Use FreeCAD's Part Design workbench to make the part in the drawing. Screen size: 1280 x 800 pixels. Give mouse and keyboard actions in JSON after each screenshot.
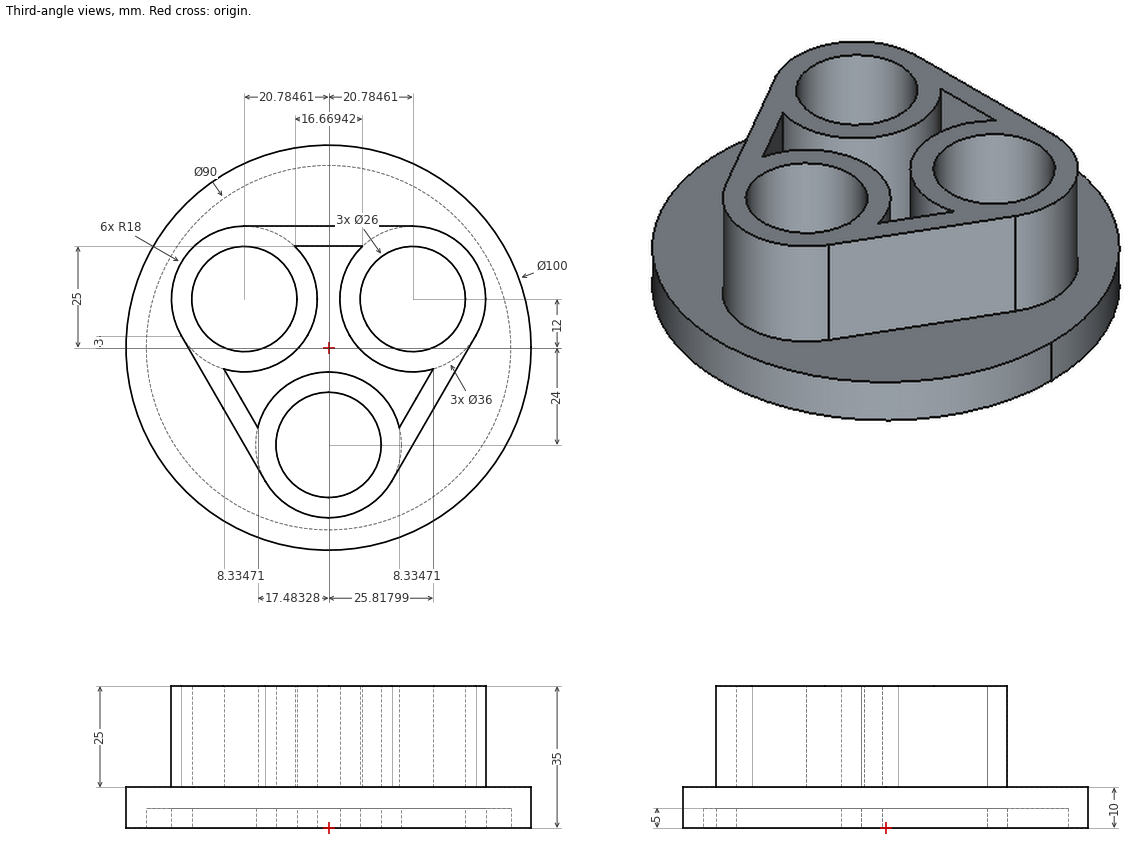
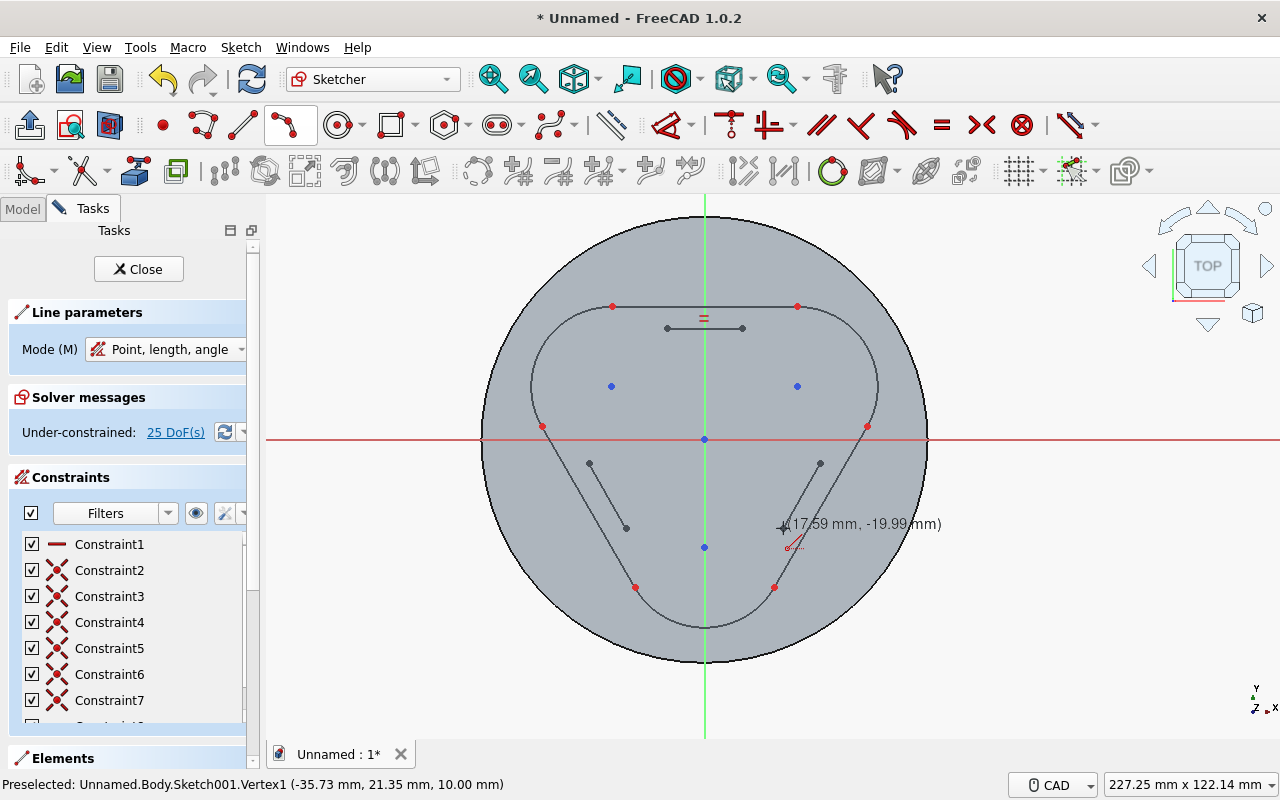
{"action": "left_click", "coordinate": [284, 126]}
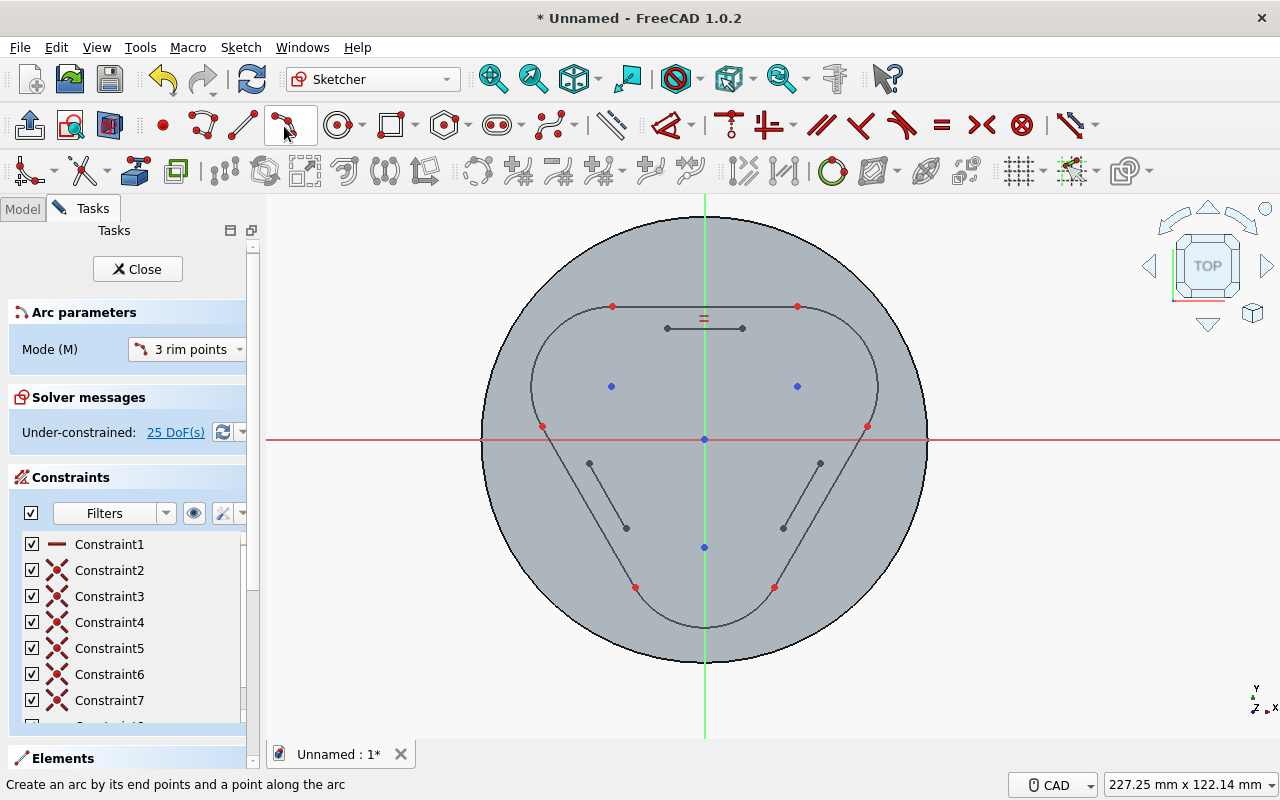
{"action": "left_click", "coordinate": [589, 464]}
{"action": "left_click", "coordinate": [667, 329]}
{"action": "left_click", "coordinate": [689, 407]}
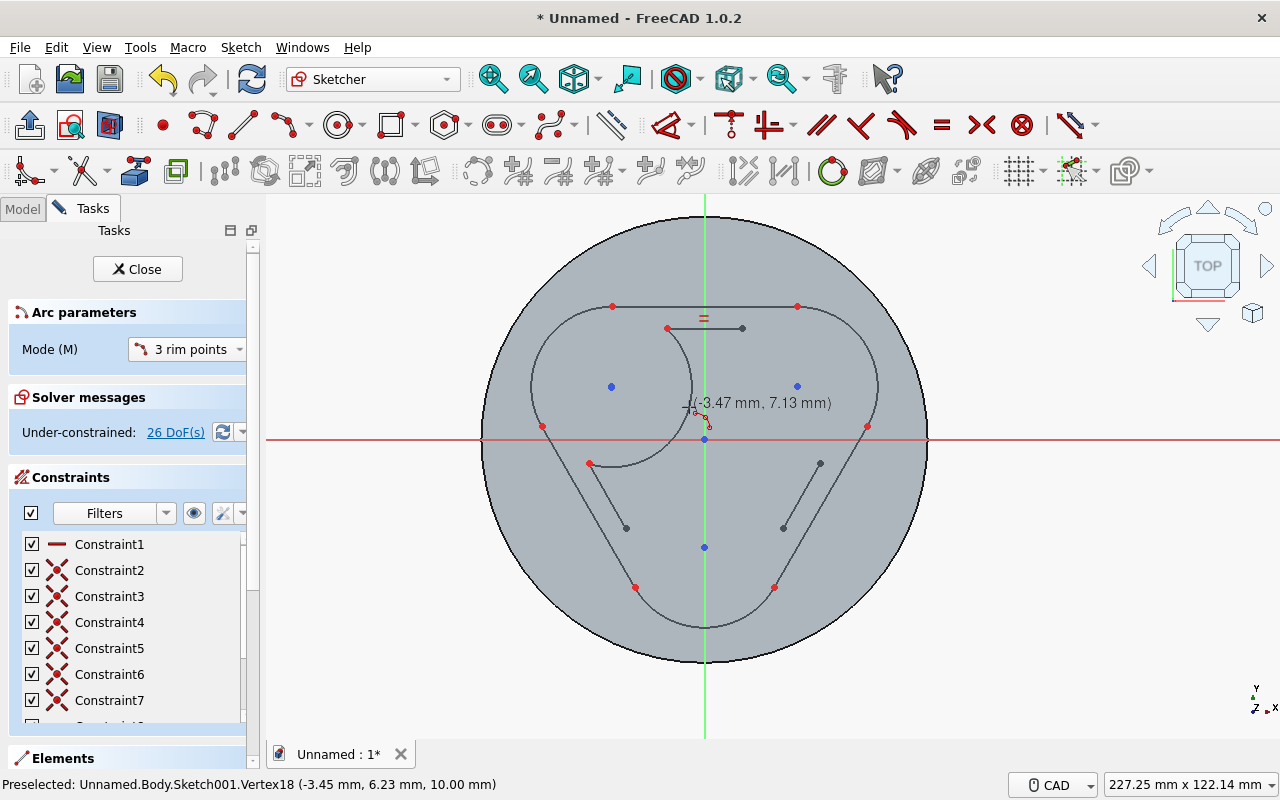
{"action": "left_click", "coordinate": [742, 329]}
{"action": "left_click", "coordinate": [820, 464]}
{"action": "left_click", "coordinate": [720, 407]}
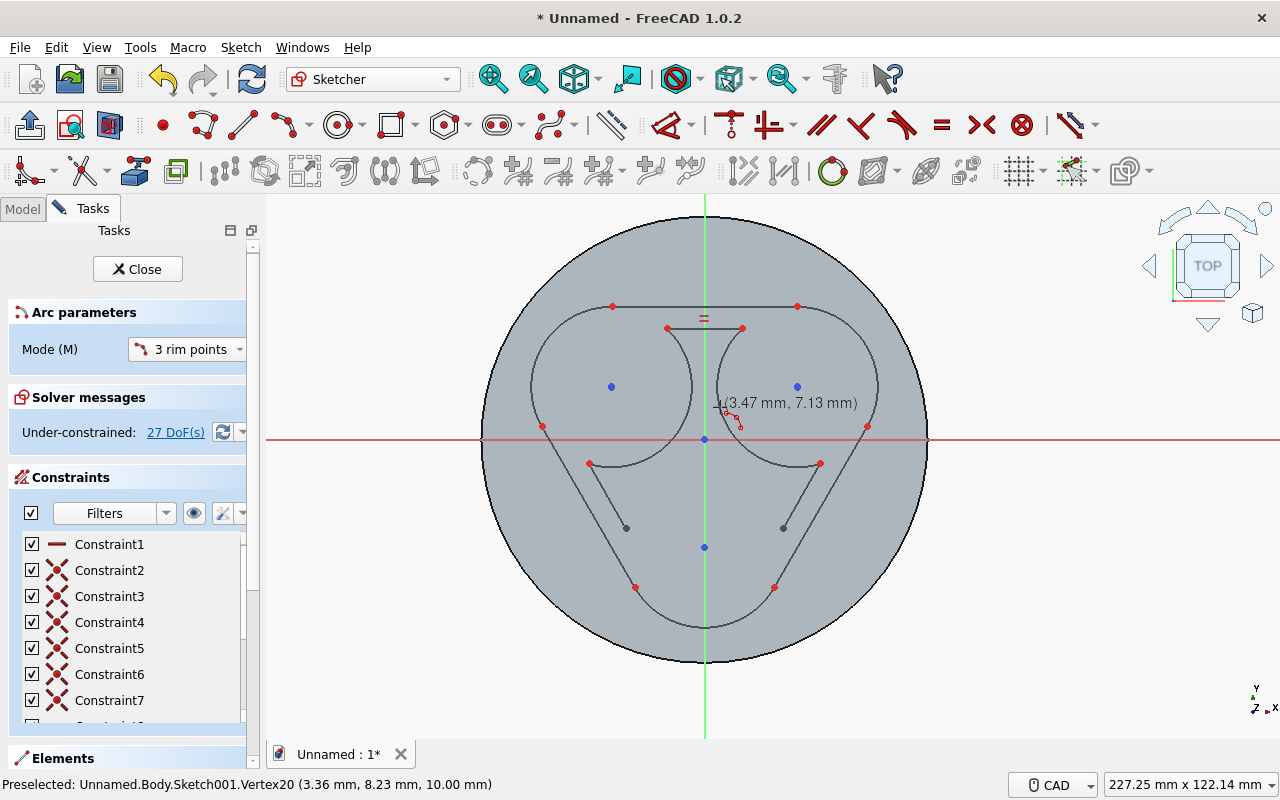
{"action": "left_click", "coordinate": [783, 529]}
{"action": "left_click", "coordinate": [626, 529]}
{"action": "left_click", "coordinate": [726, 469]}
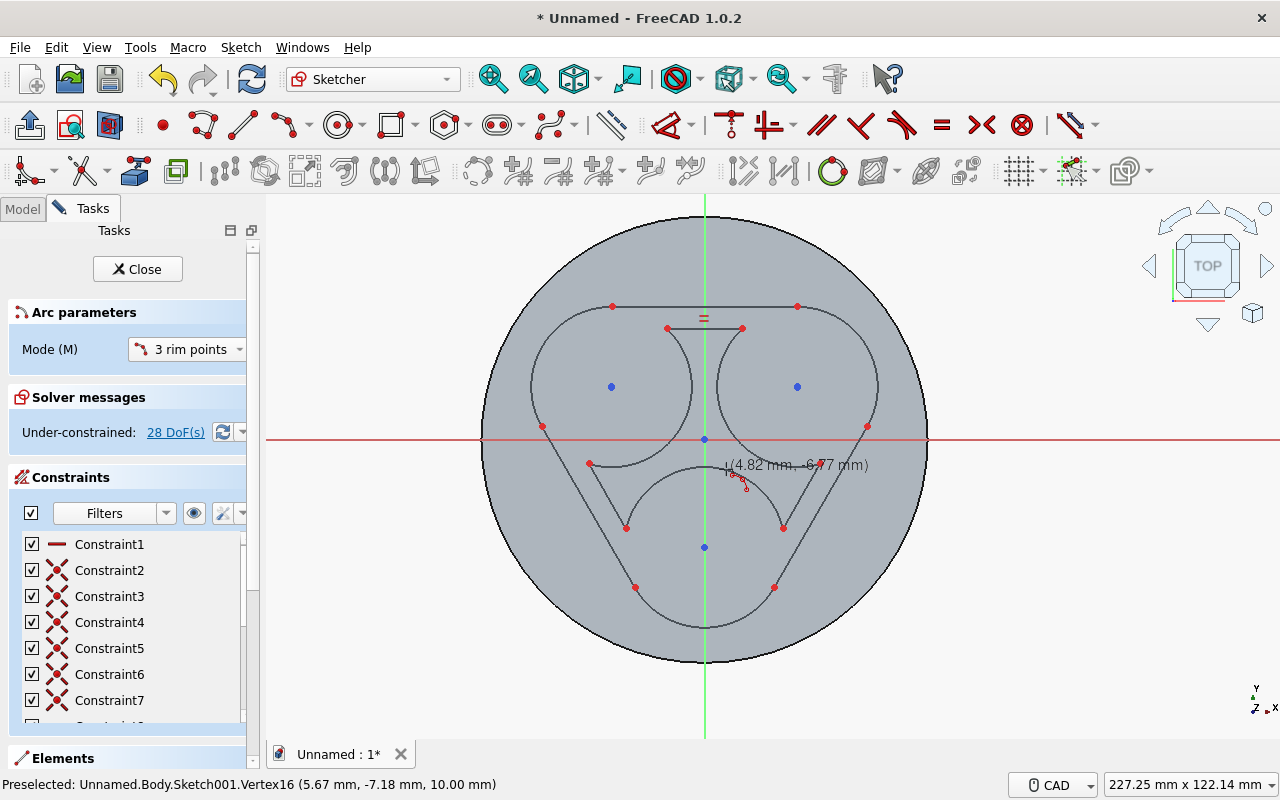
{"action": "left_click", "coordinate": [338, 126]}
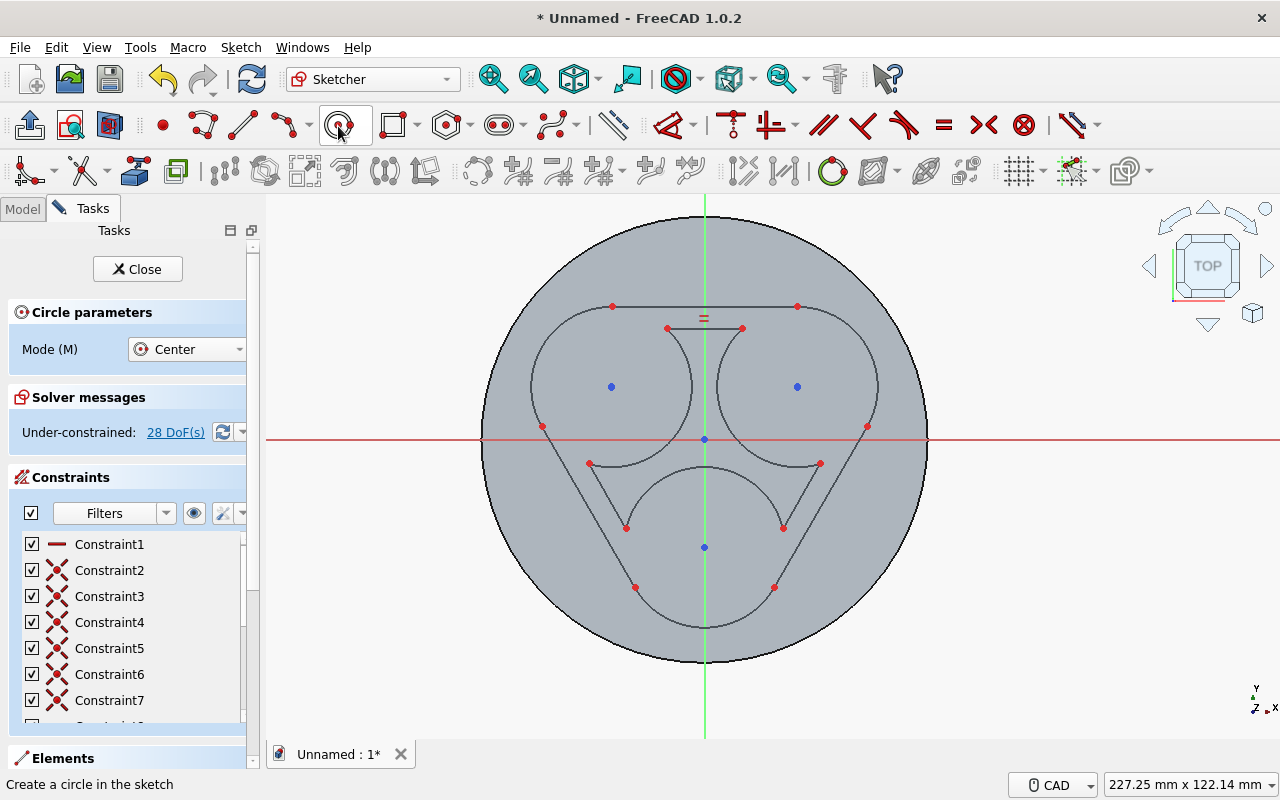
{"action": "left_click", "coordinate": [797, 386]}
{"action": "left_click", "coordinate": [838, 345]}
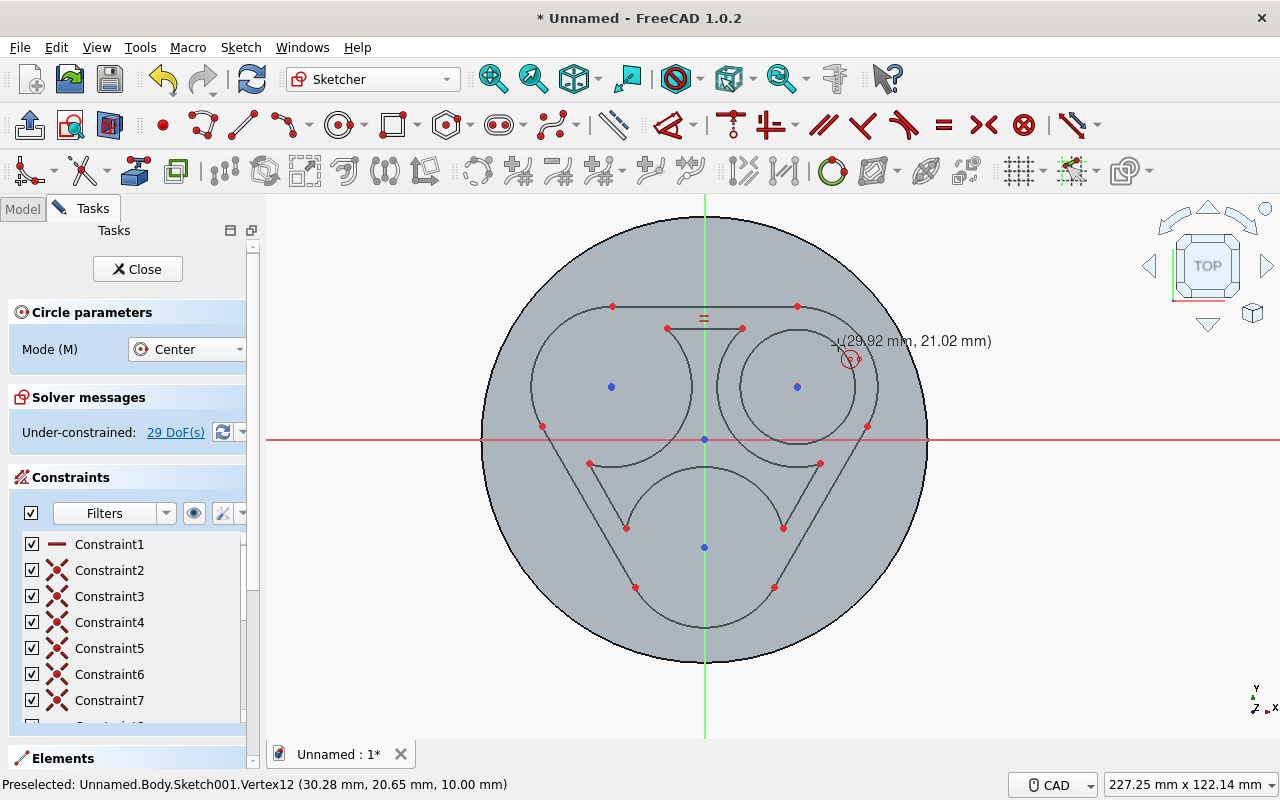
{"action": "left_click", "coordinate": [705, 547]}
{"action": "left_click", "coordinate": [746, 506]}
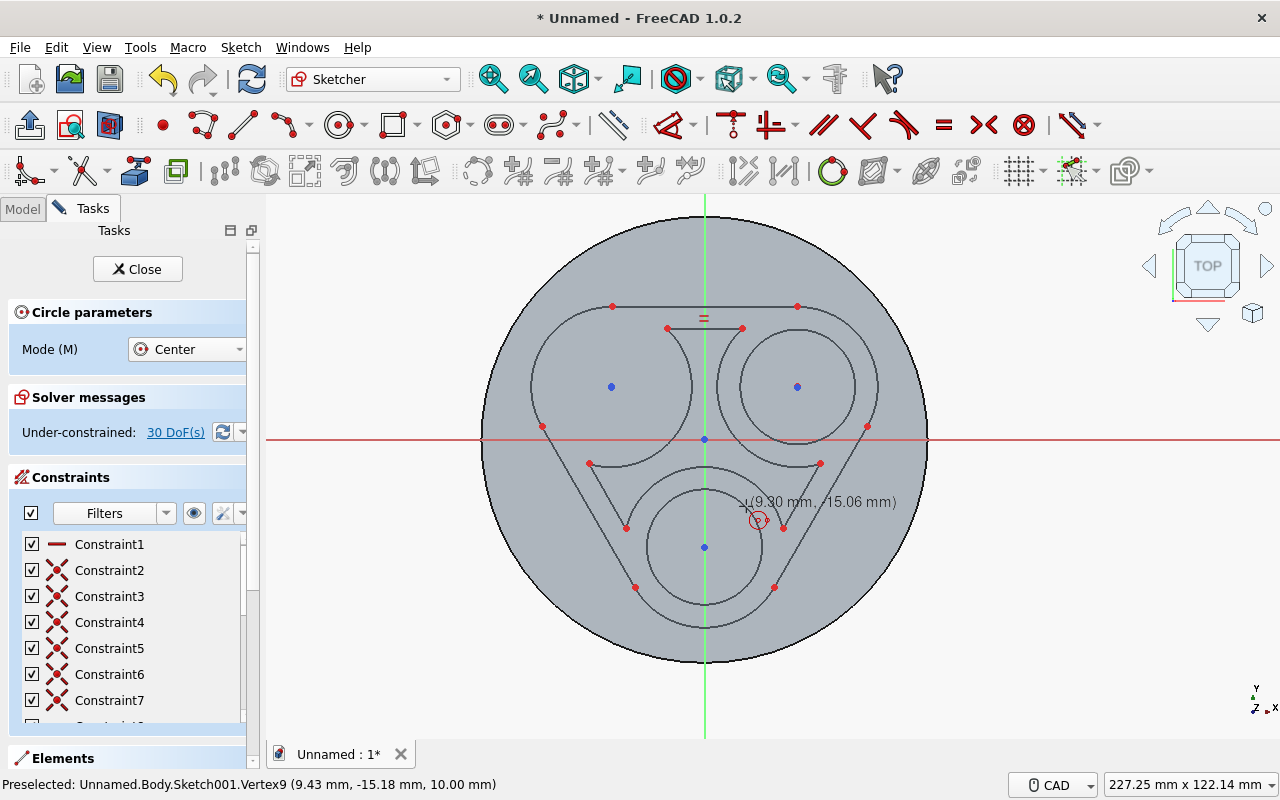
{"action": "left_click", "coordinate": [612, 386]}
{"action": "left_click", "coordinate": [653, 345]}
{"action": "key", "text": "Escape"}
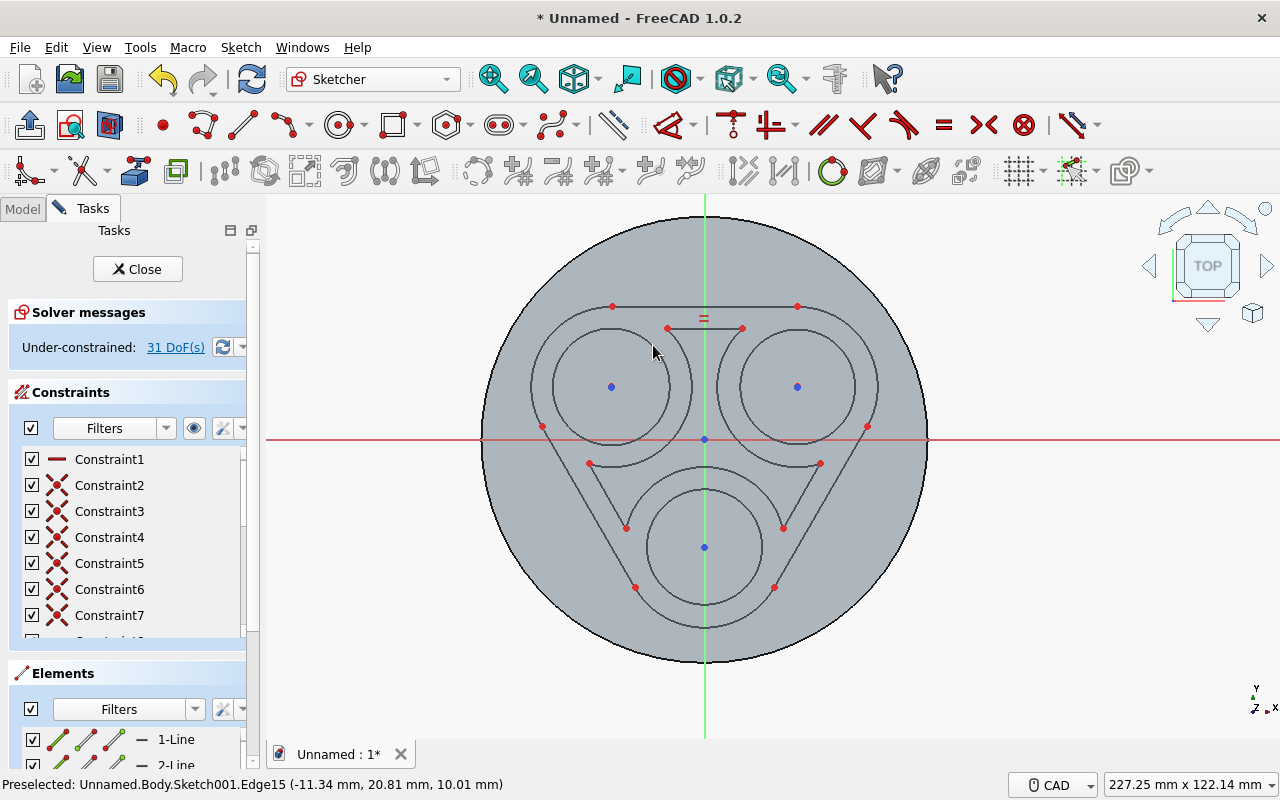
{"action": "left_click", "coordinate": [570, 475]}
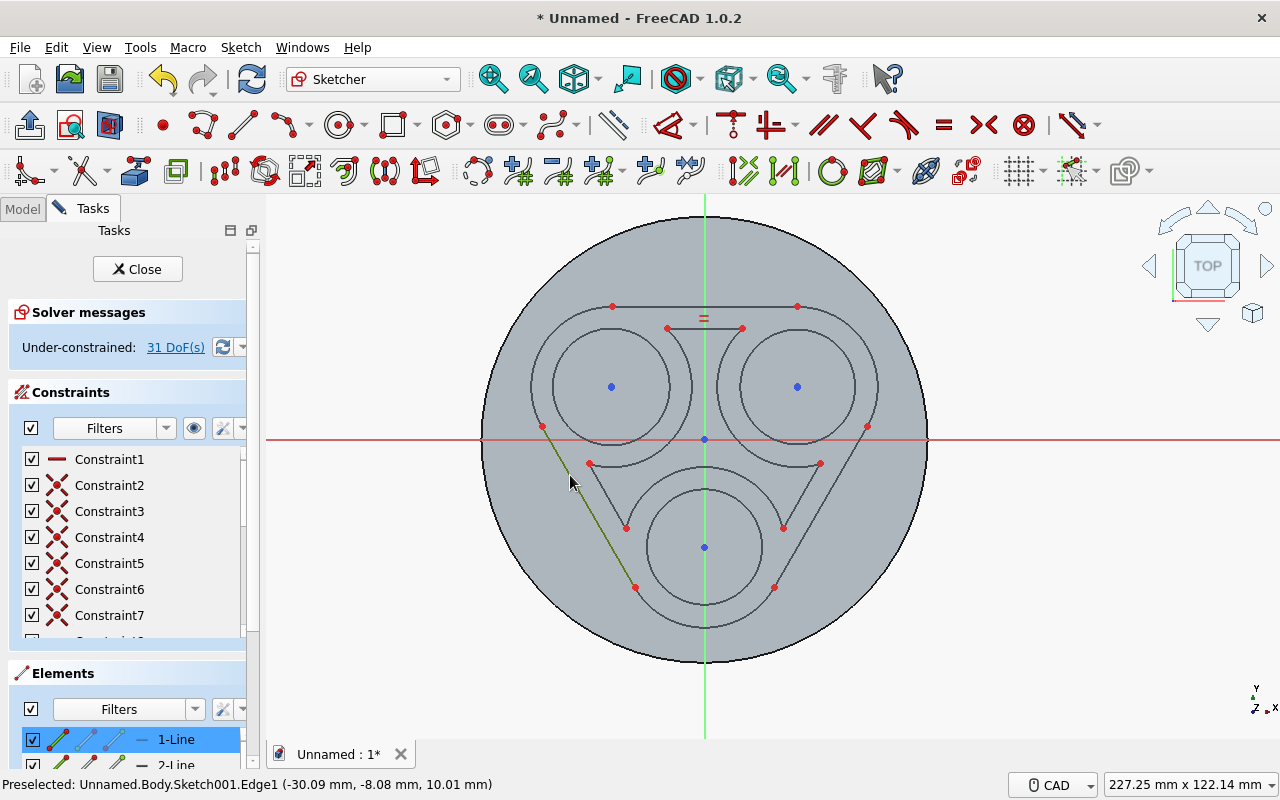
{"action": "left_click", "coordinate": [672, 621]}